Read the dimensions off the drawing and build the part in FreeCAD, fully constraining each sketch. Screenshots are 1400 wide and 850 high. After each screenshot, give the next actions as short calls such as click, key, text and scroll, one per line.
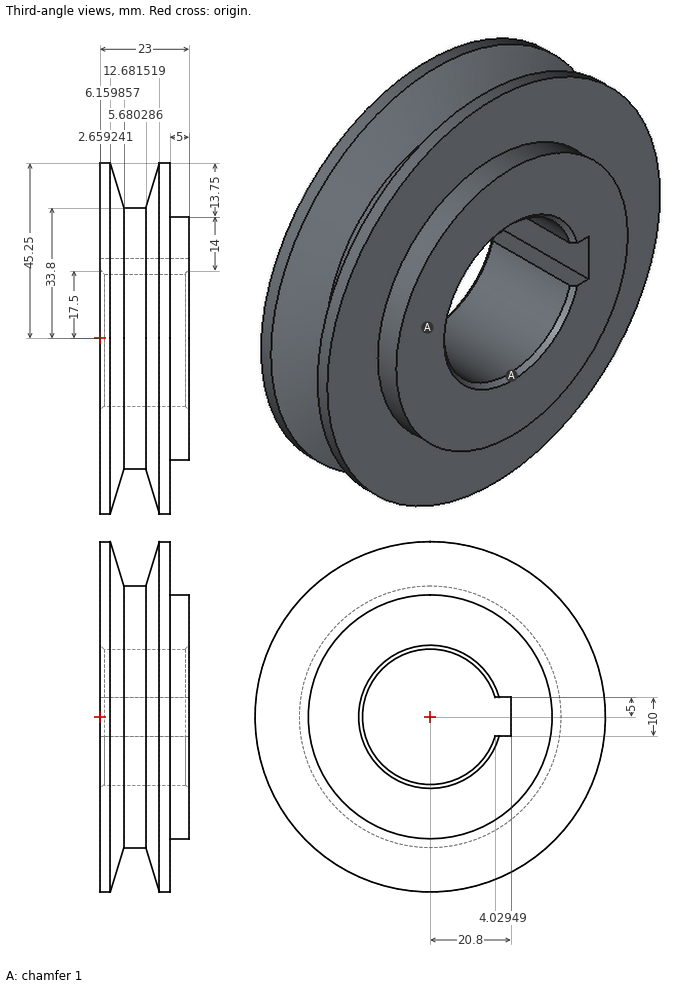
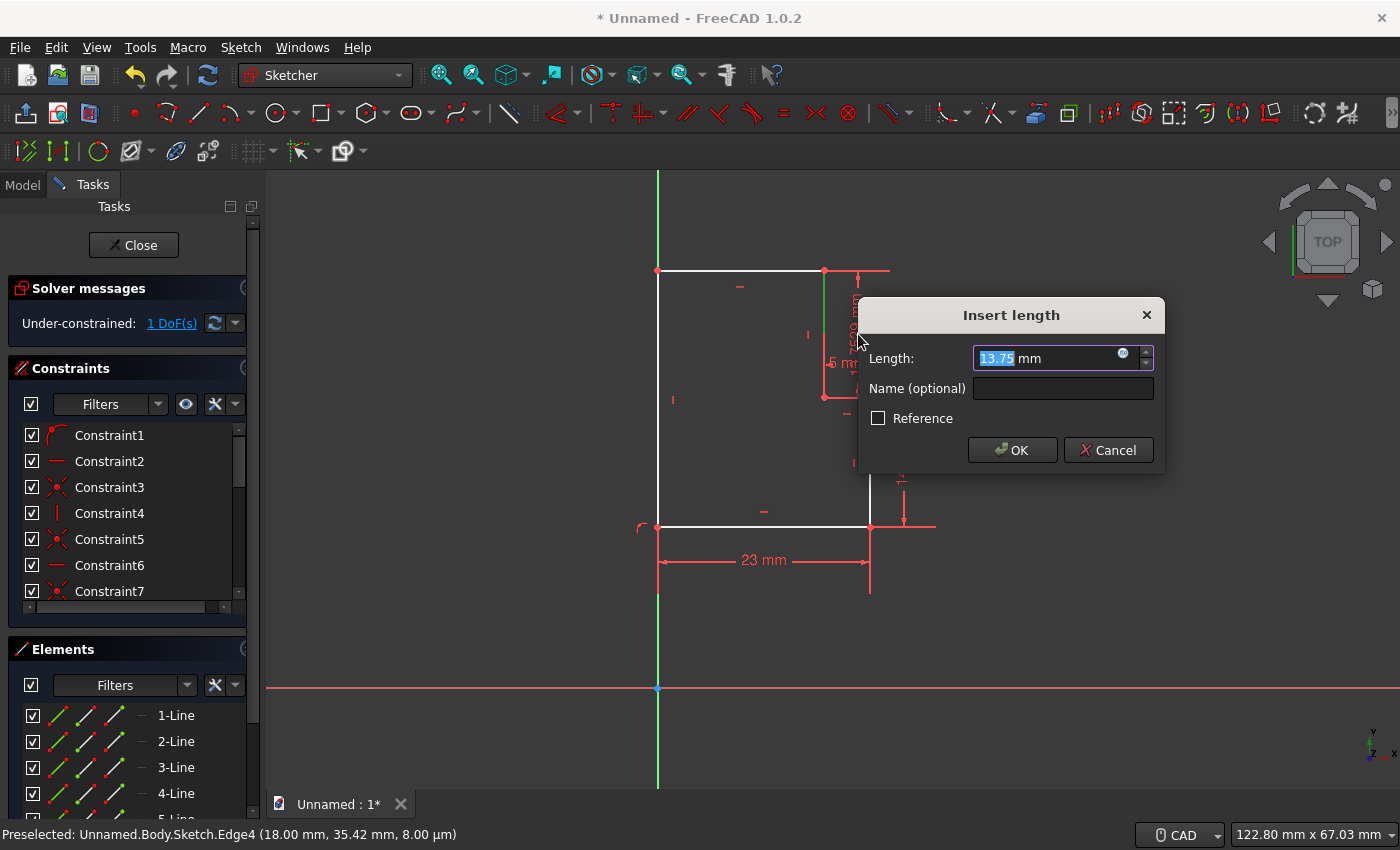
text(13.75)
key(Return)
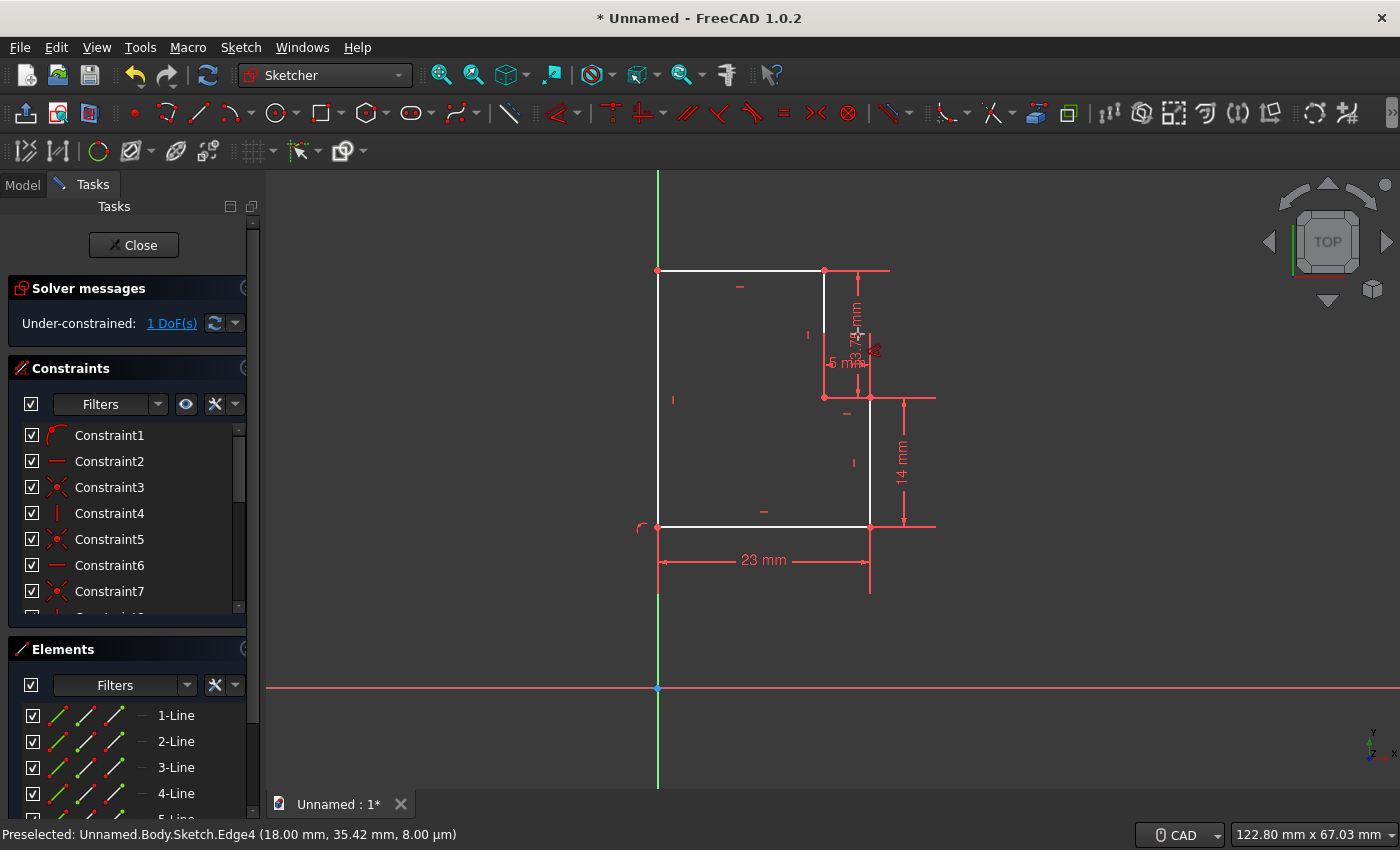
click(658, 527)
click(624, 608)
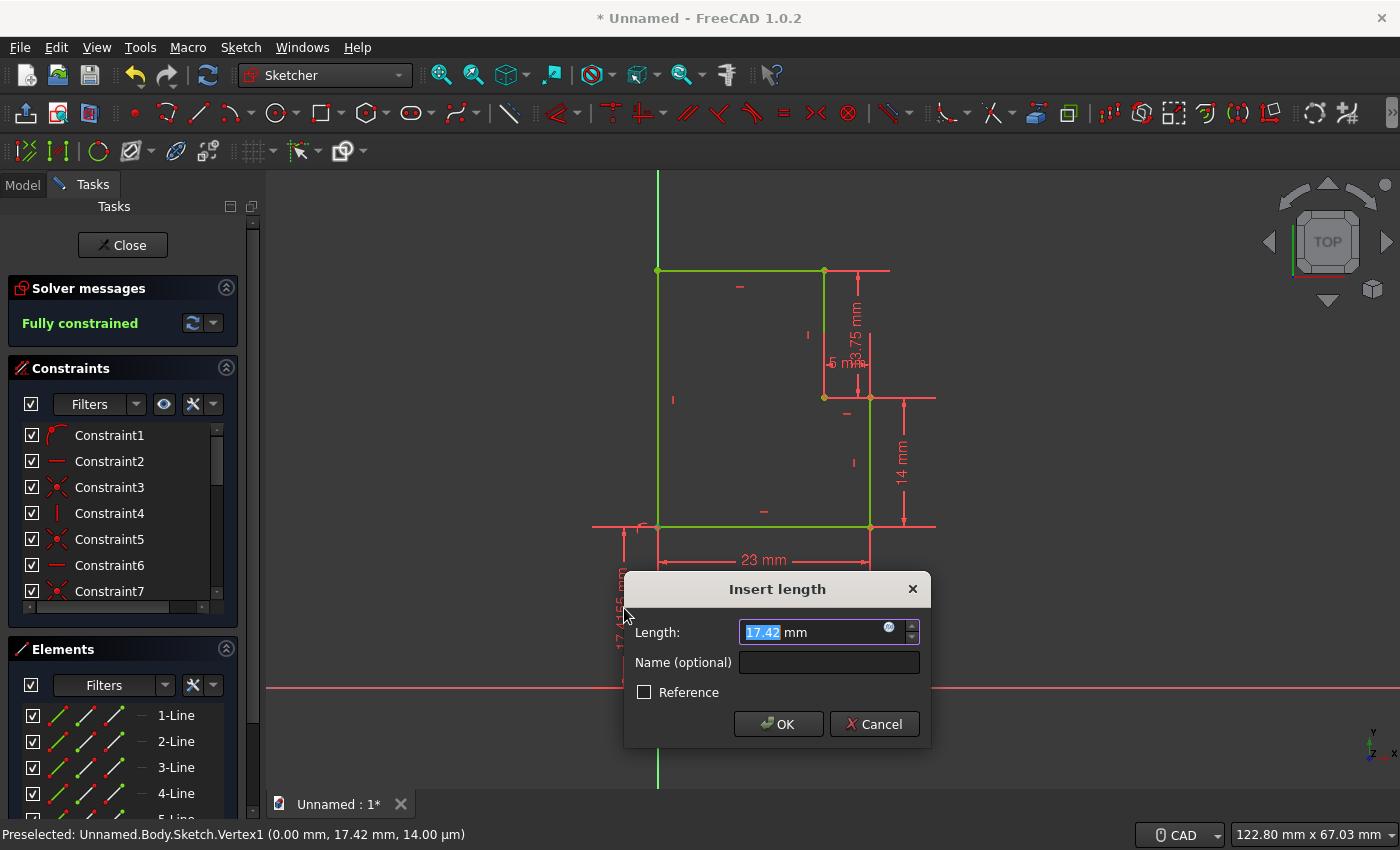
text(17.5)
key(Return)
key(Escape)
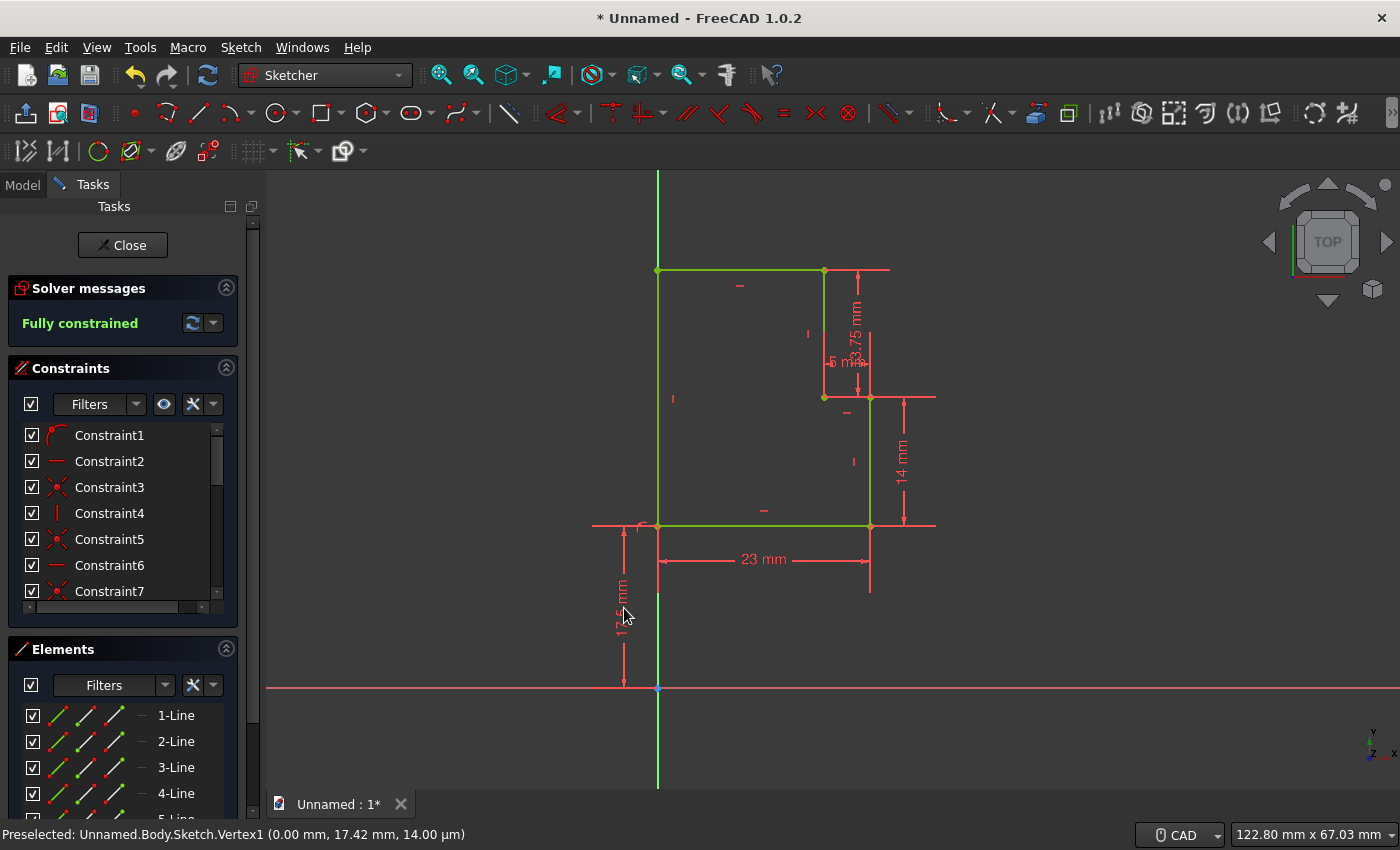
click(123, 245)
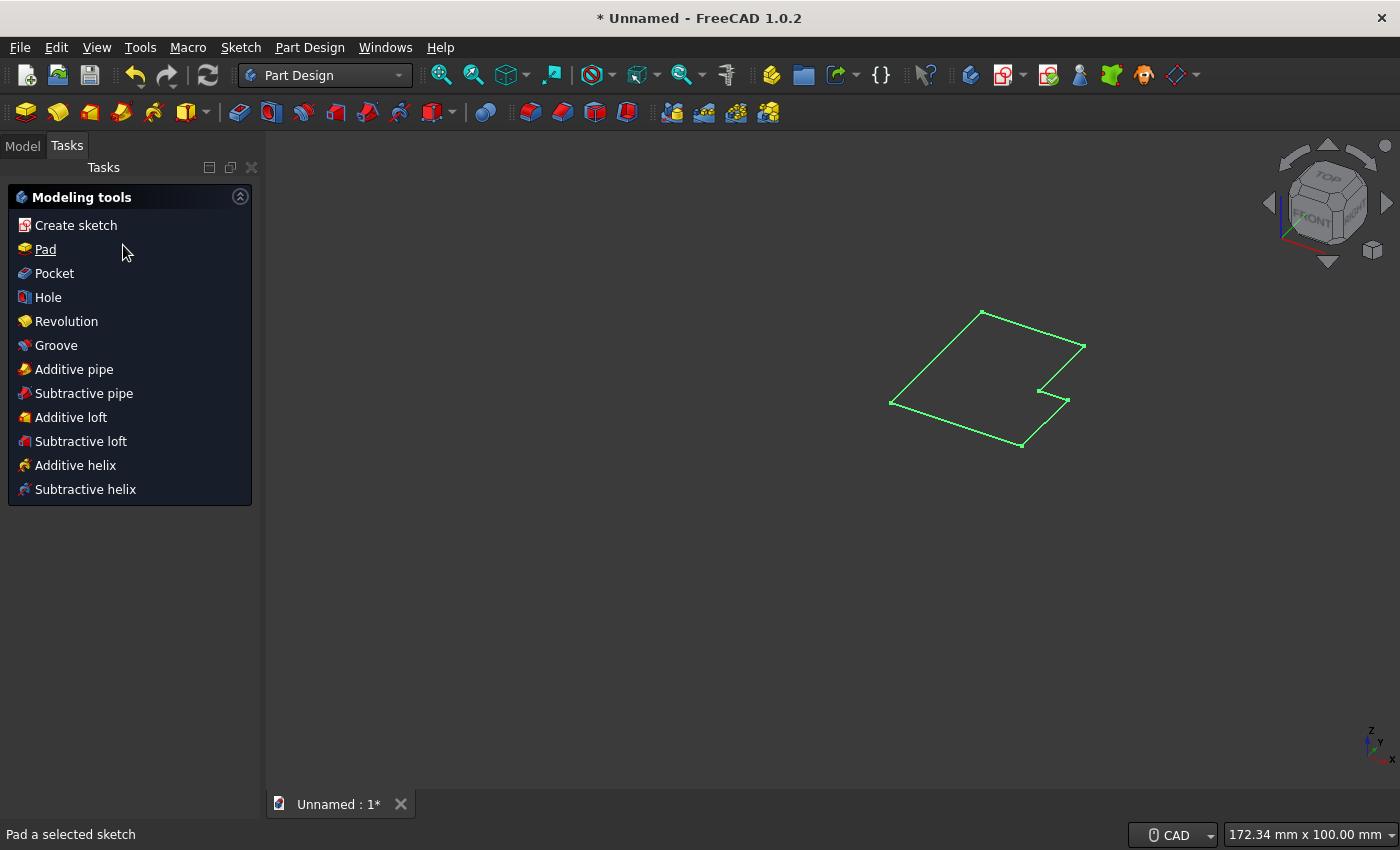
click(58, 112)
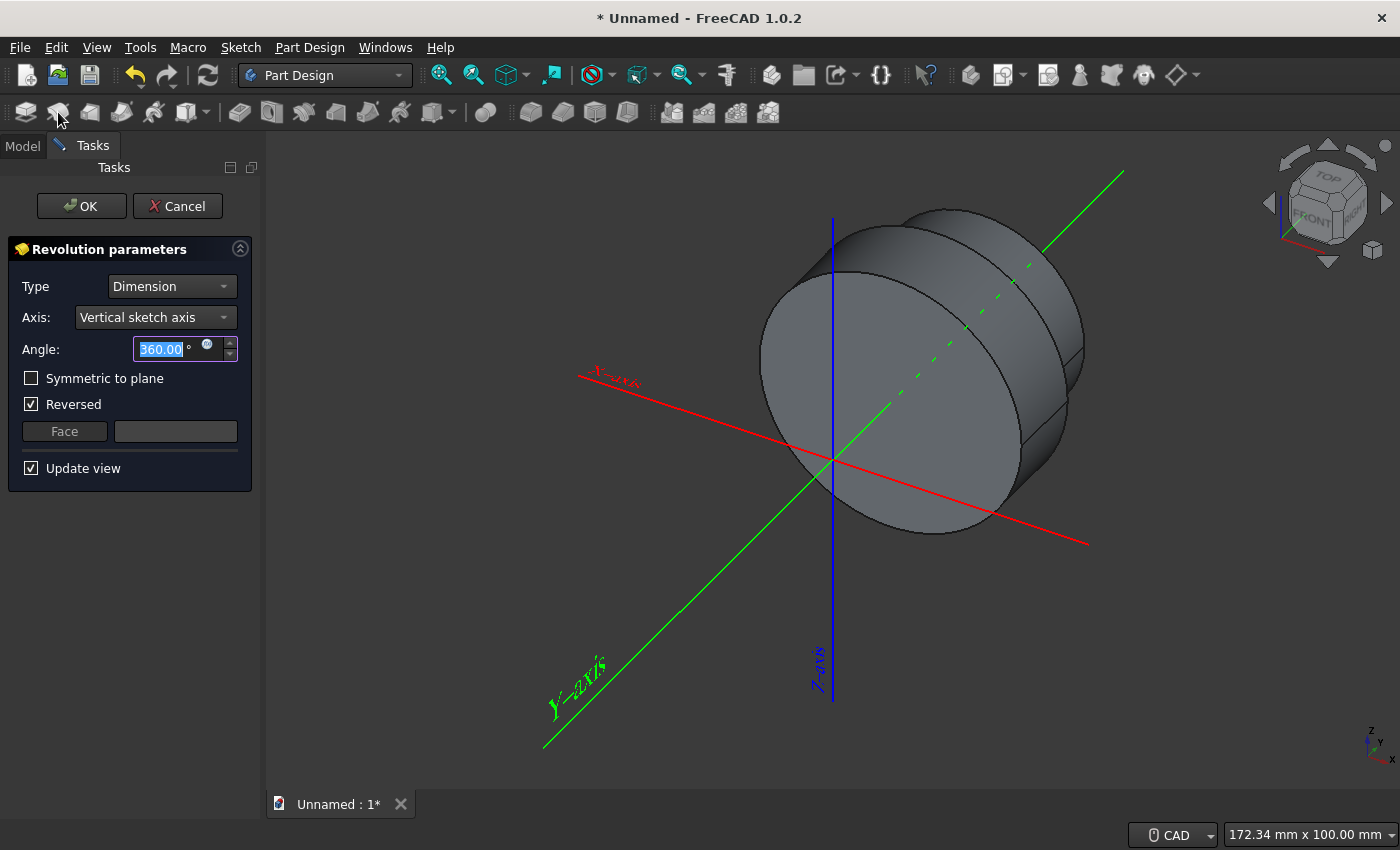
click(156, 318)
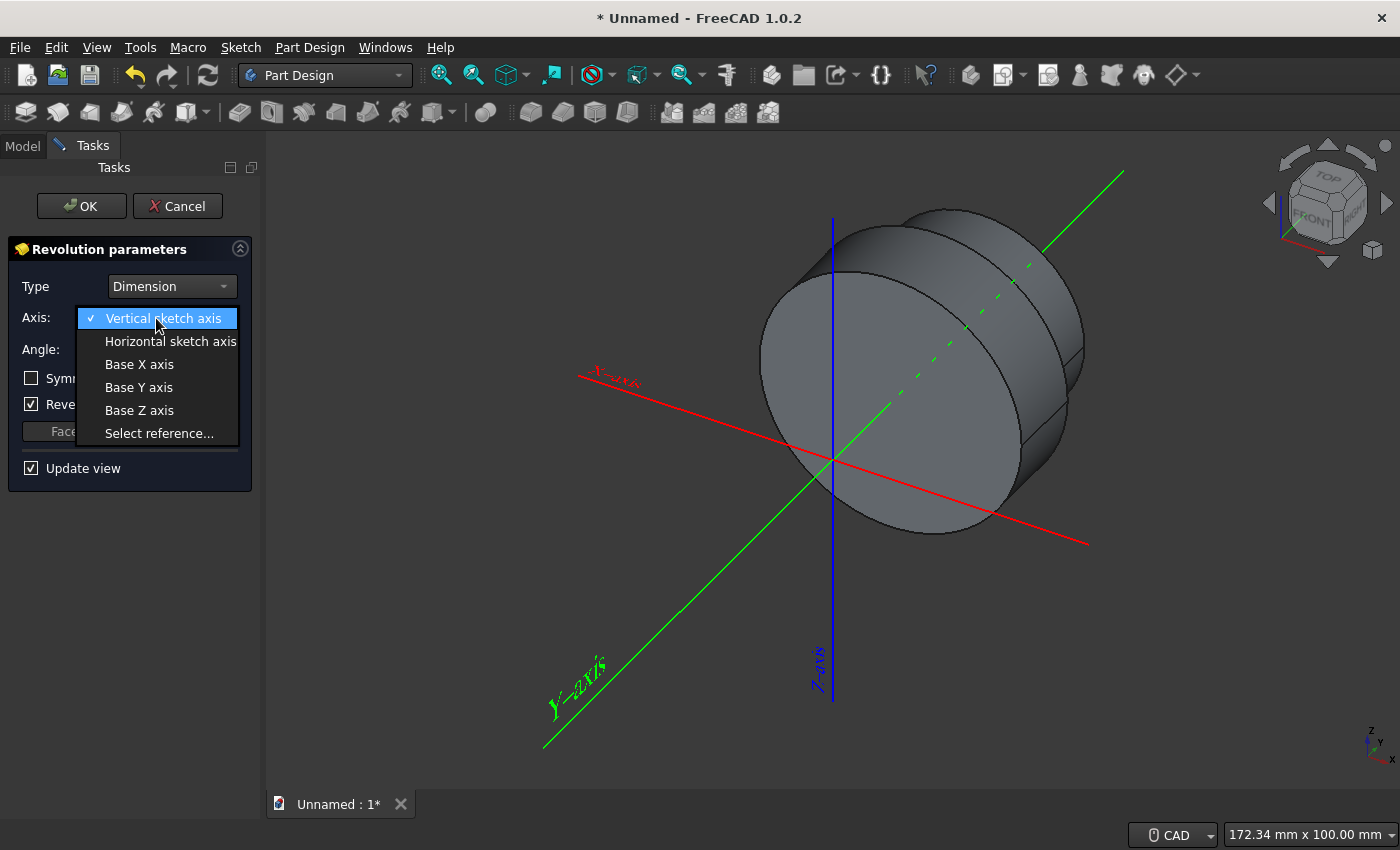
click(156, 342)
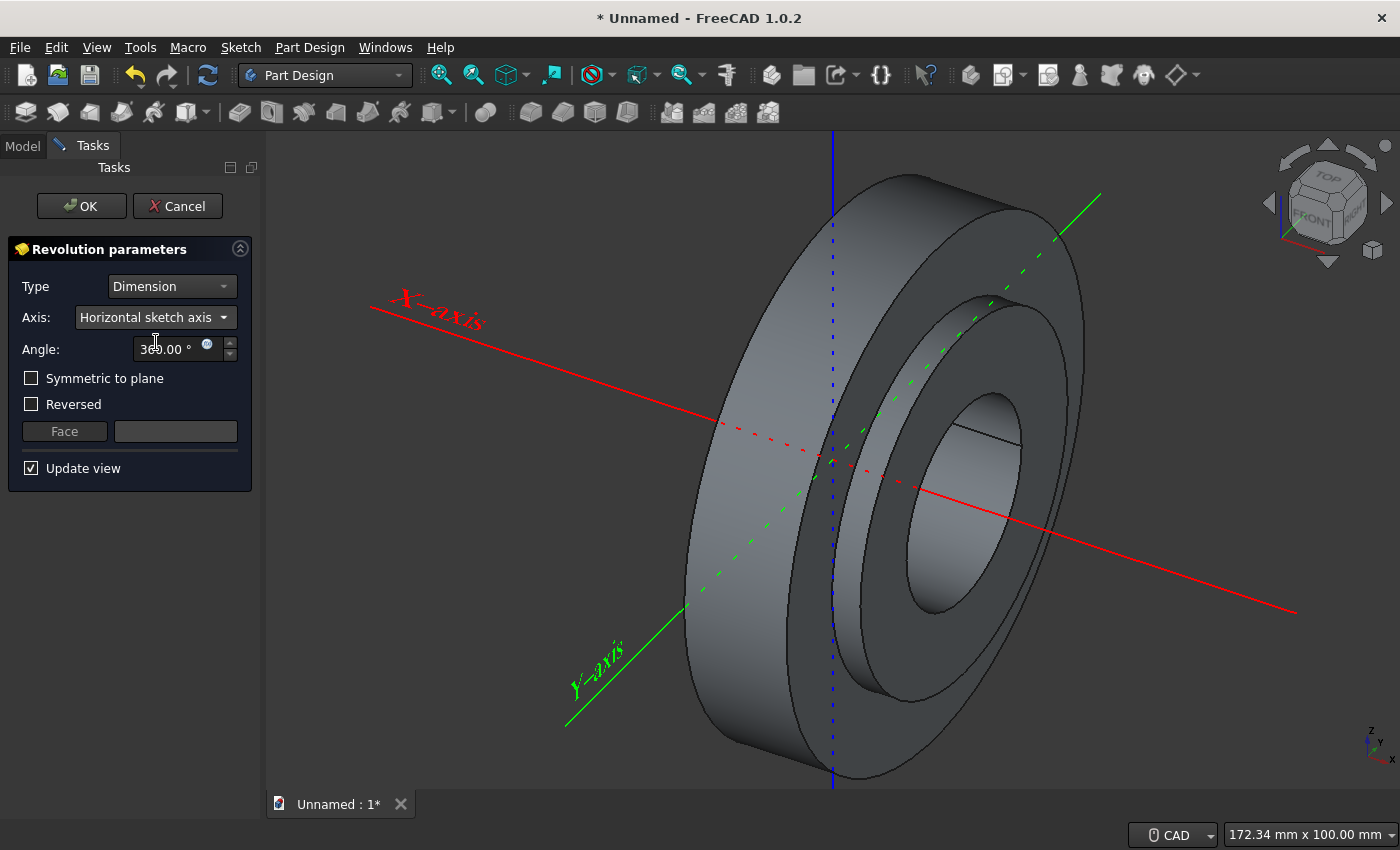
click(82, 206)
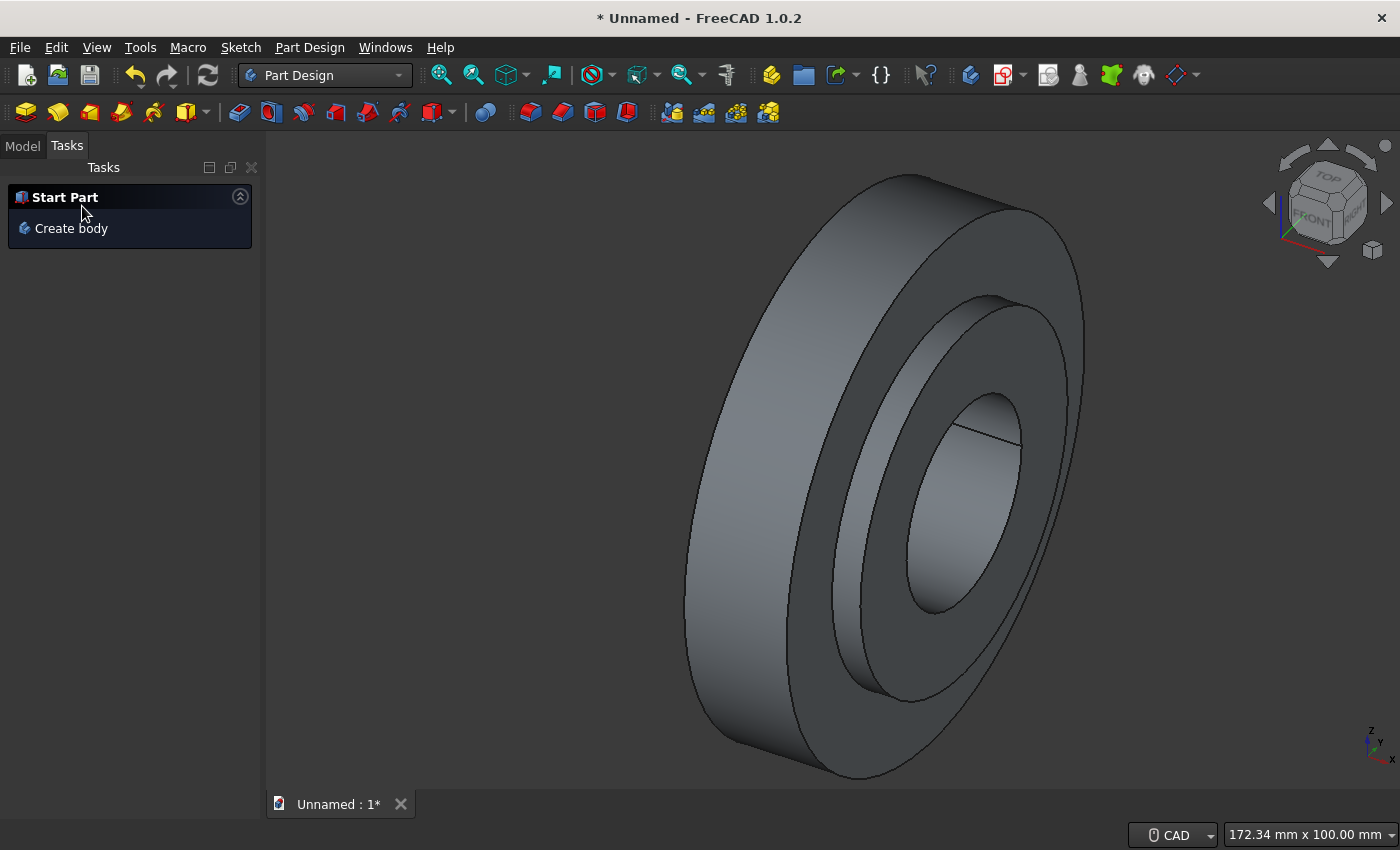
key(v)
key(f)